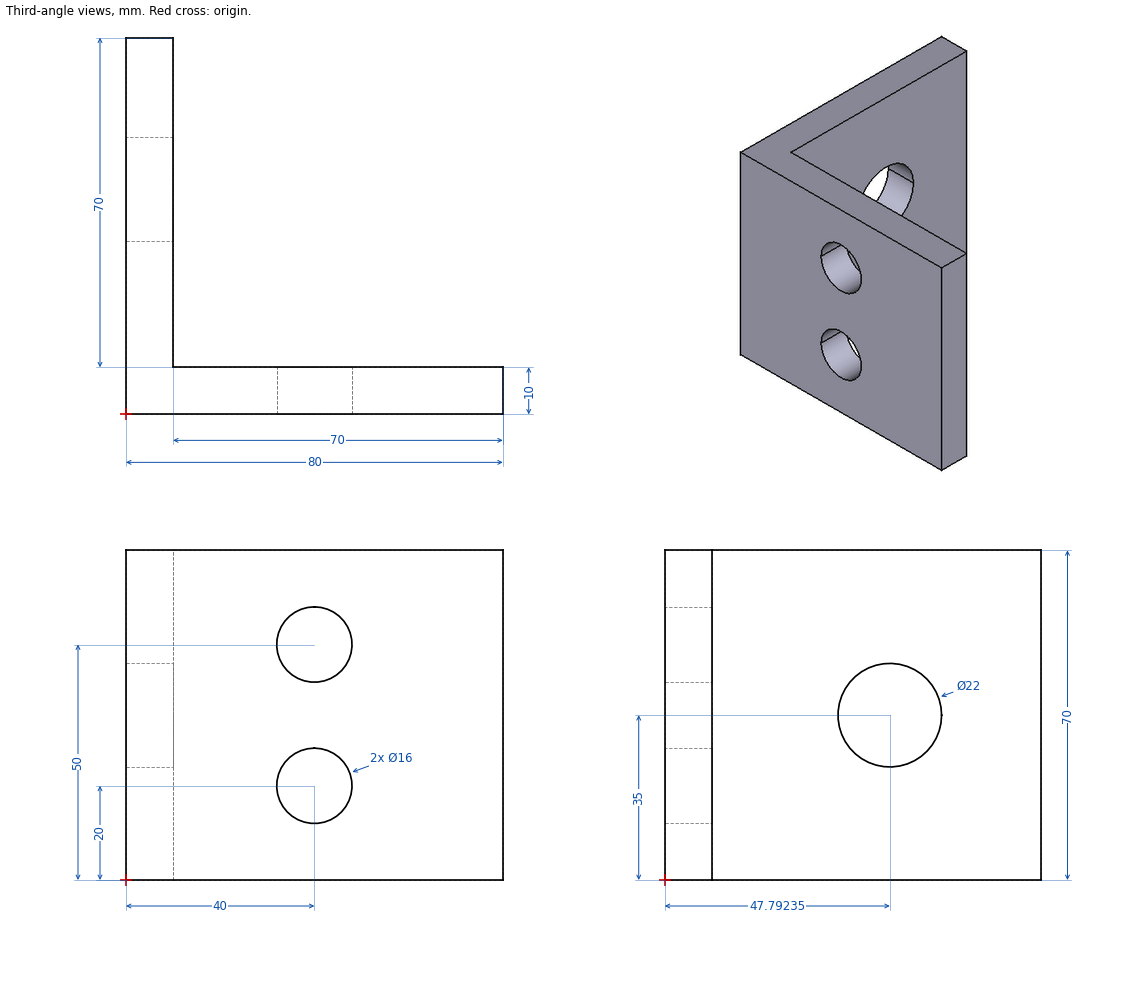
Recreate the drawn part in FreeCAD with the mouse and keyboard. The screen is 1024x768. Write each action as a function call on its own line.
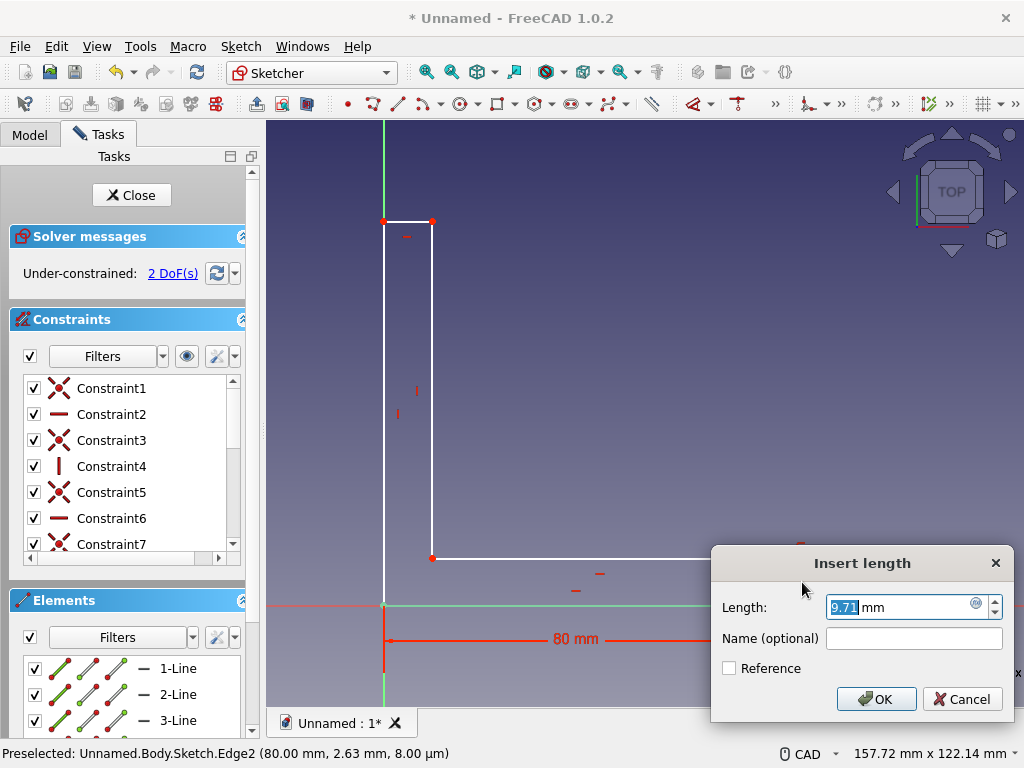
text(10)
key(Return)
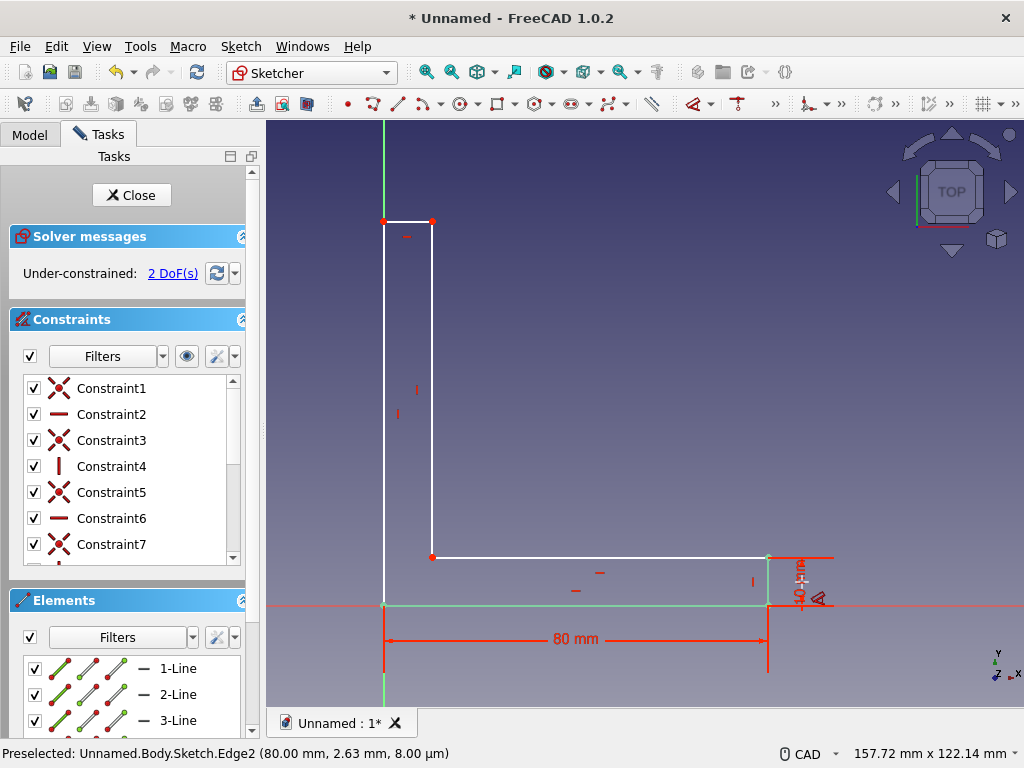
click(667, 558)
click(600, 592)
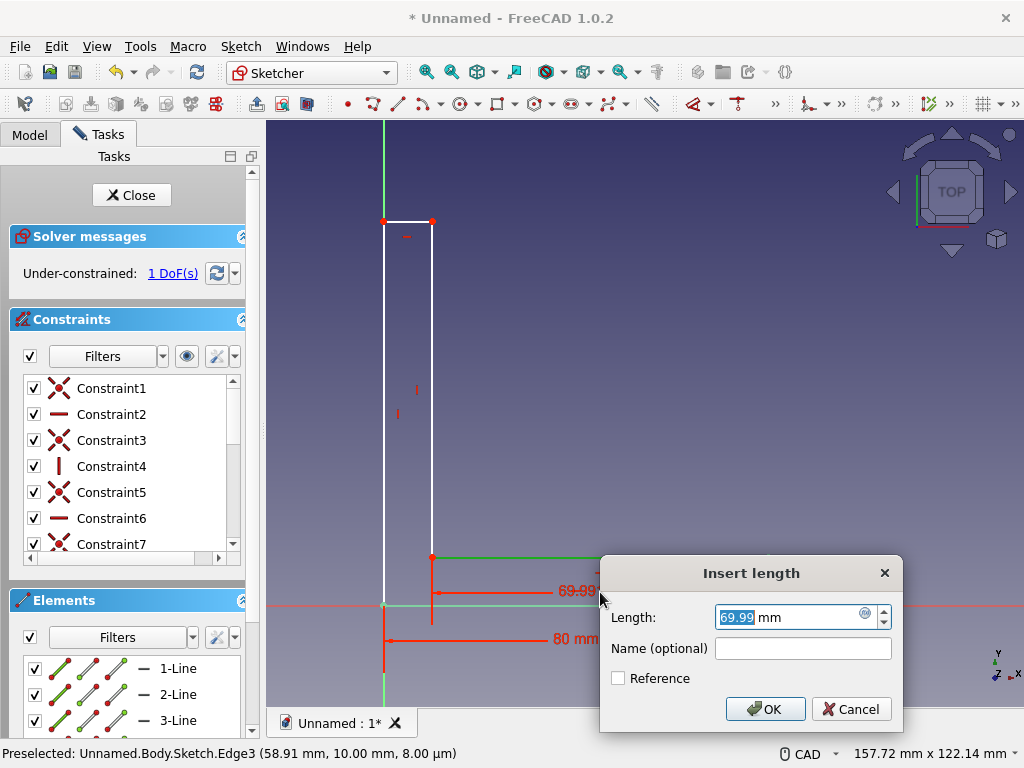
text(70)
key(Return)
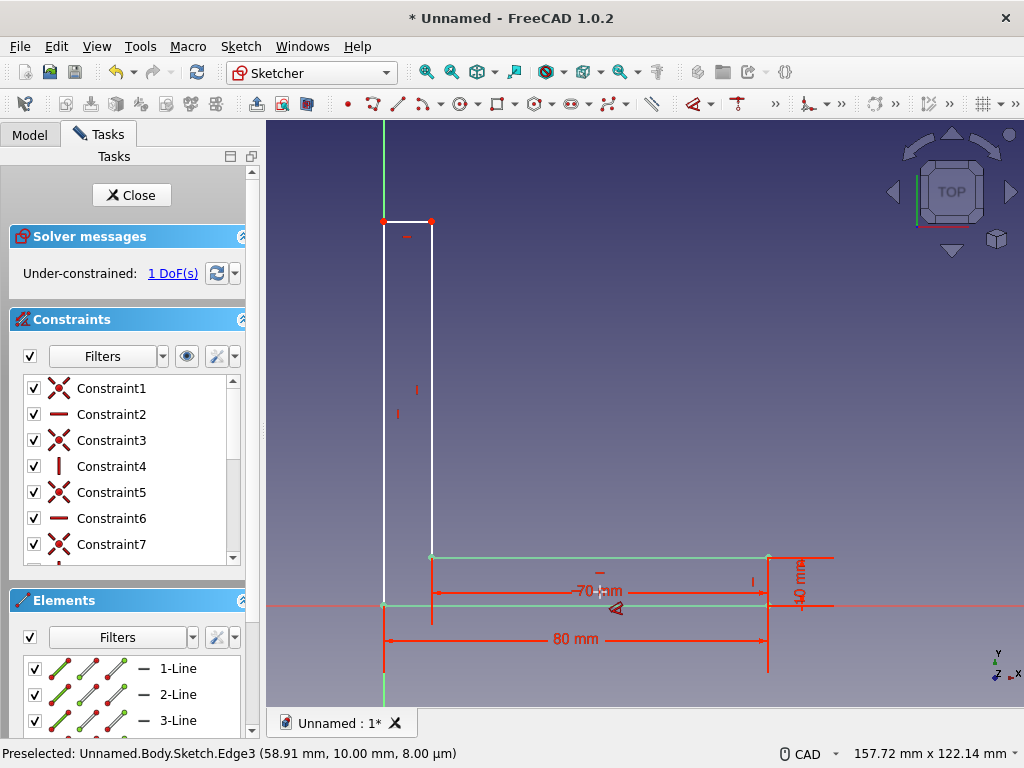
click(432, 457)
click(398, 390)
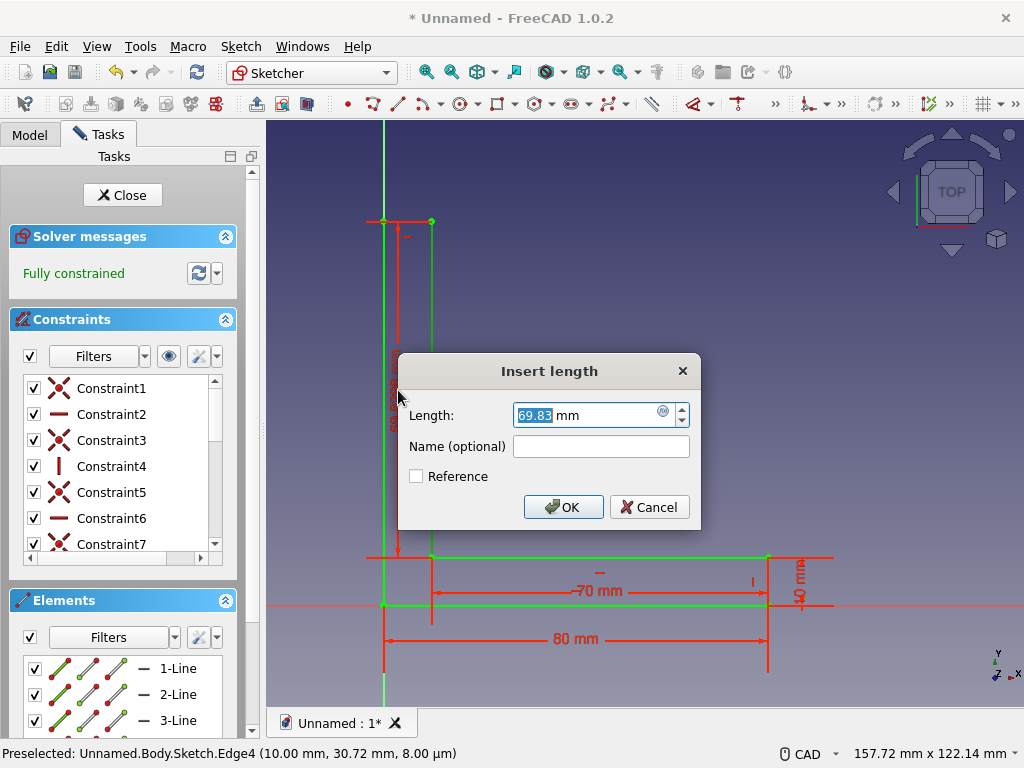
text(70)
key(Return)
key(Escape)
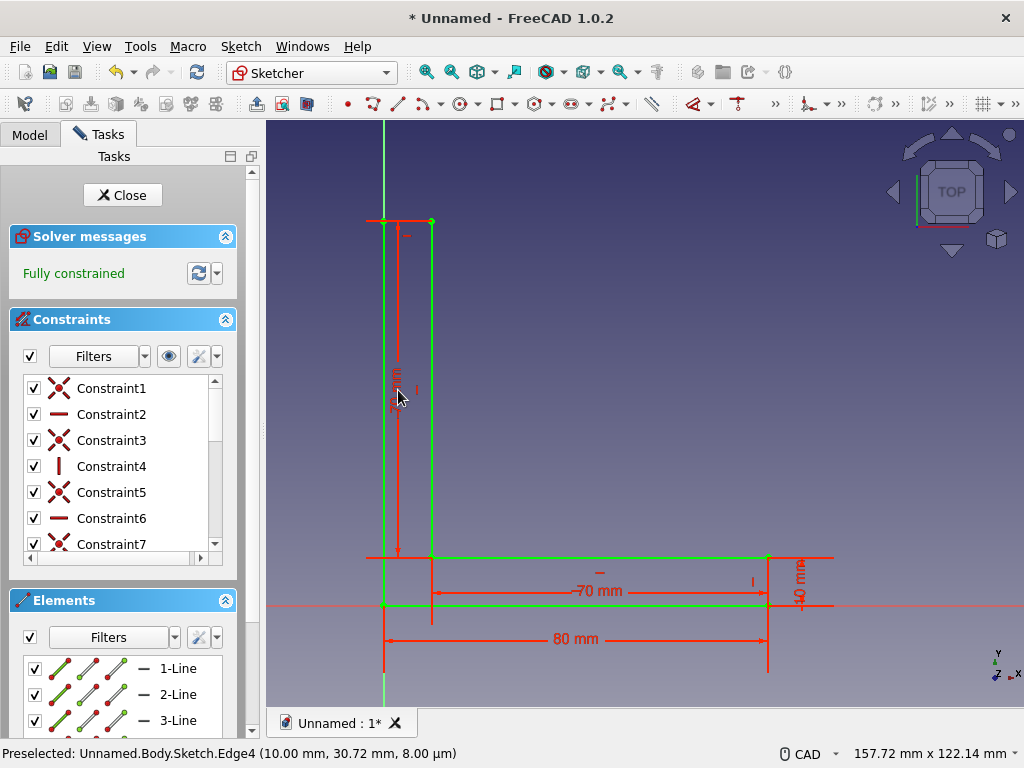
click(123, 195)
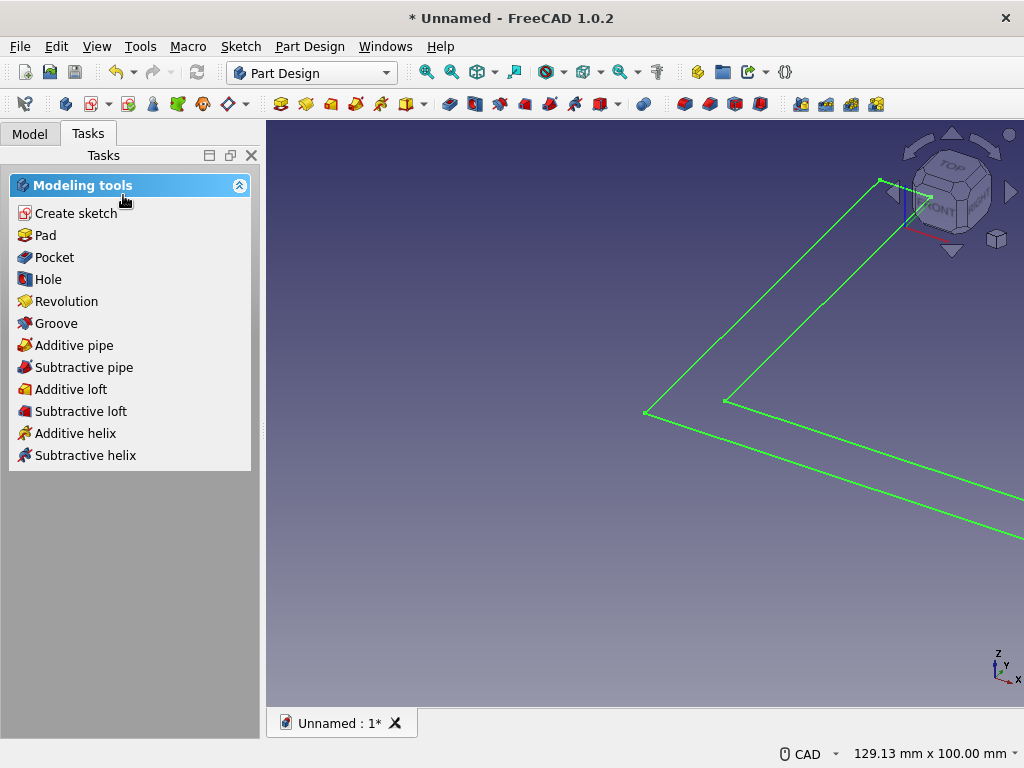
click(281, 104)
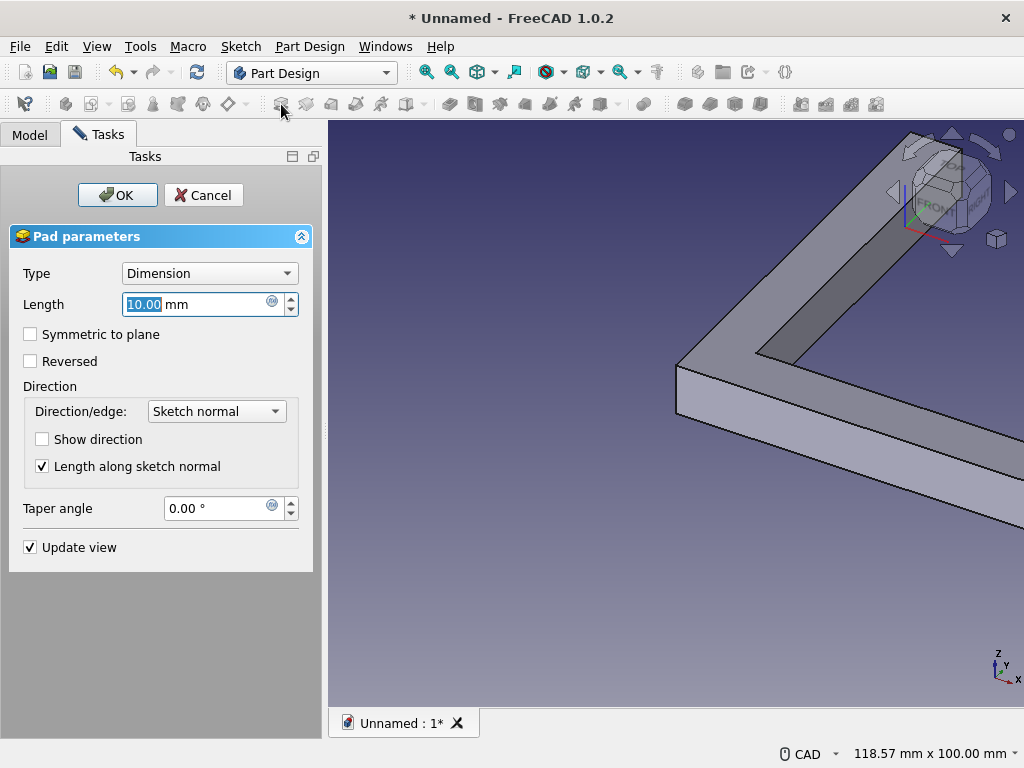
text(70)
key(Tab)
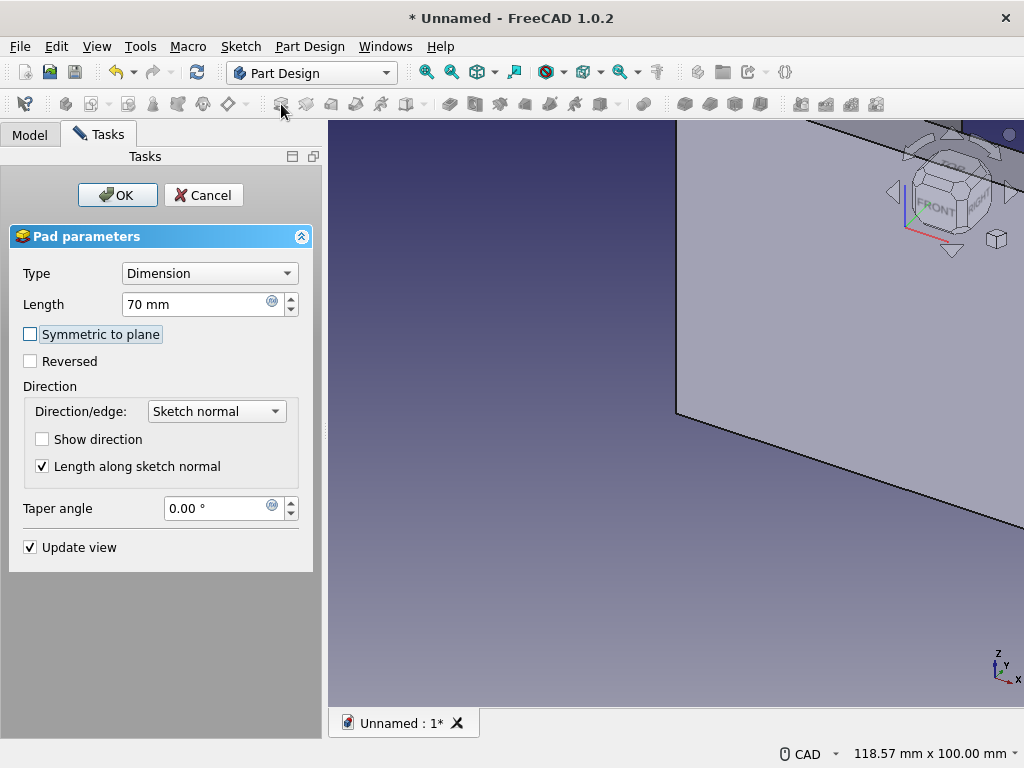
click(118, 195)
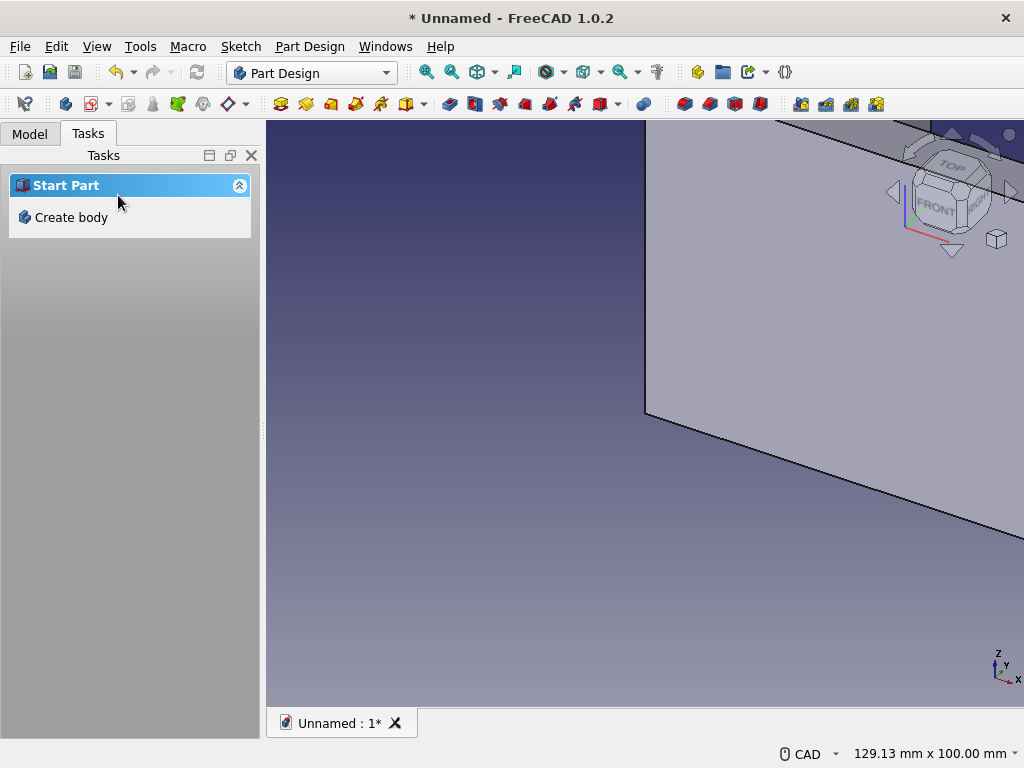
click(427, 72)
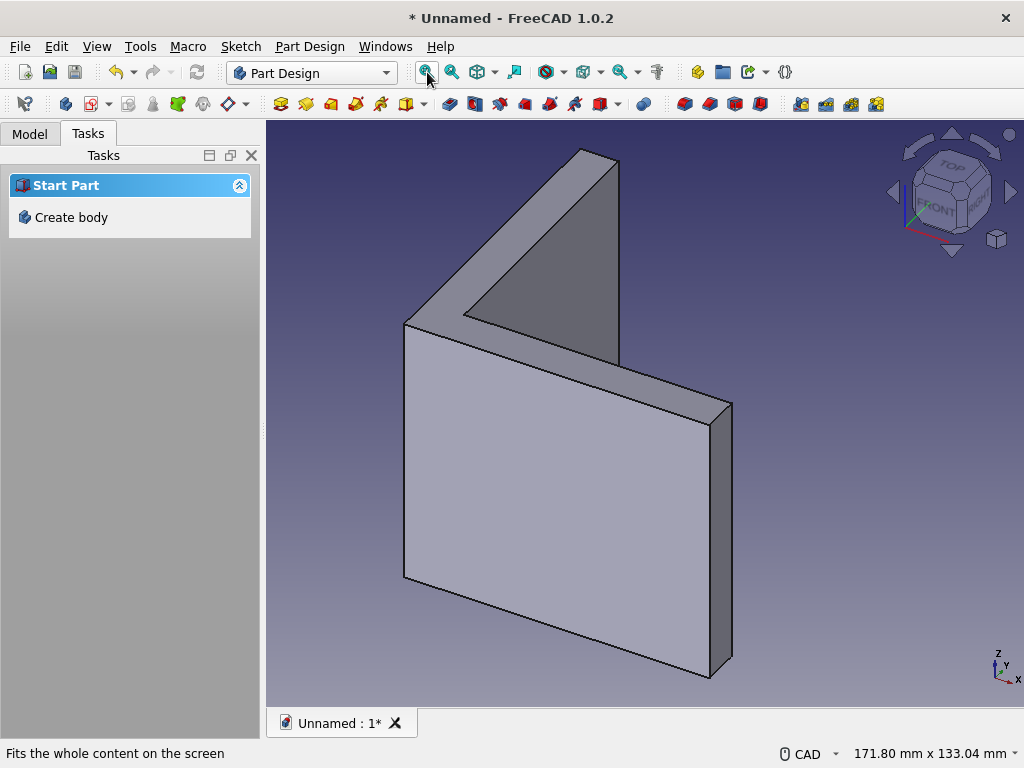
key(4)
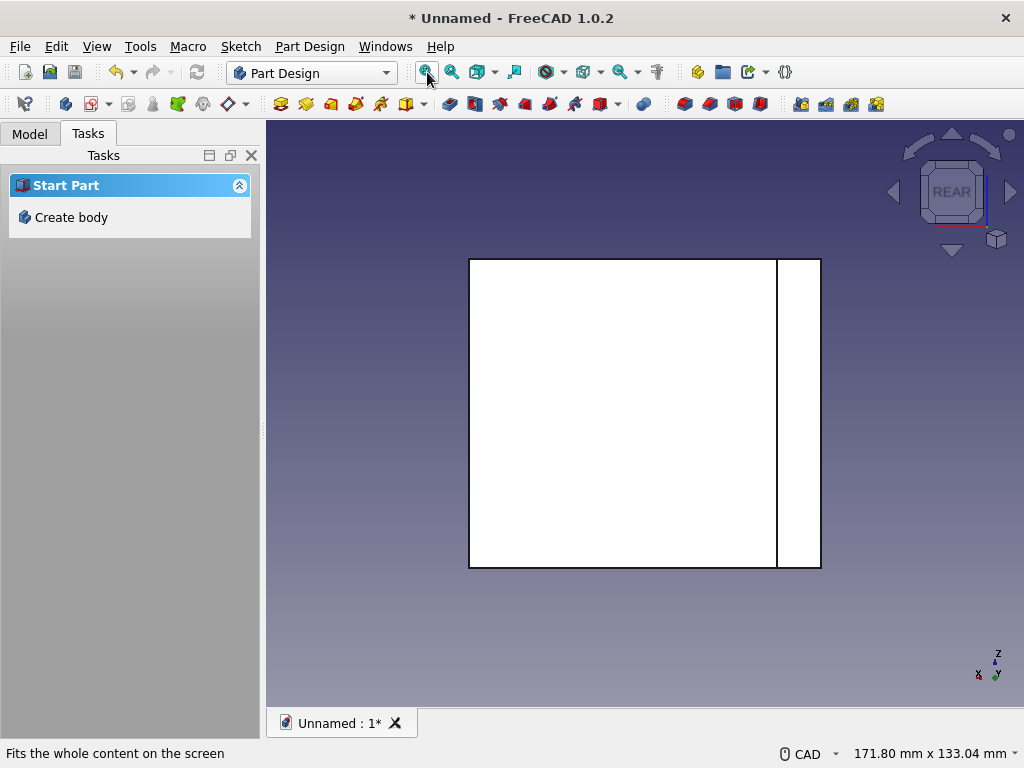
click(623, 412)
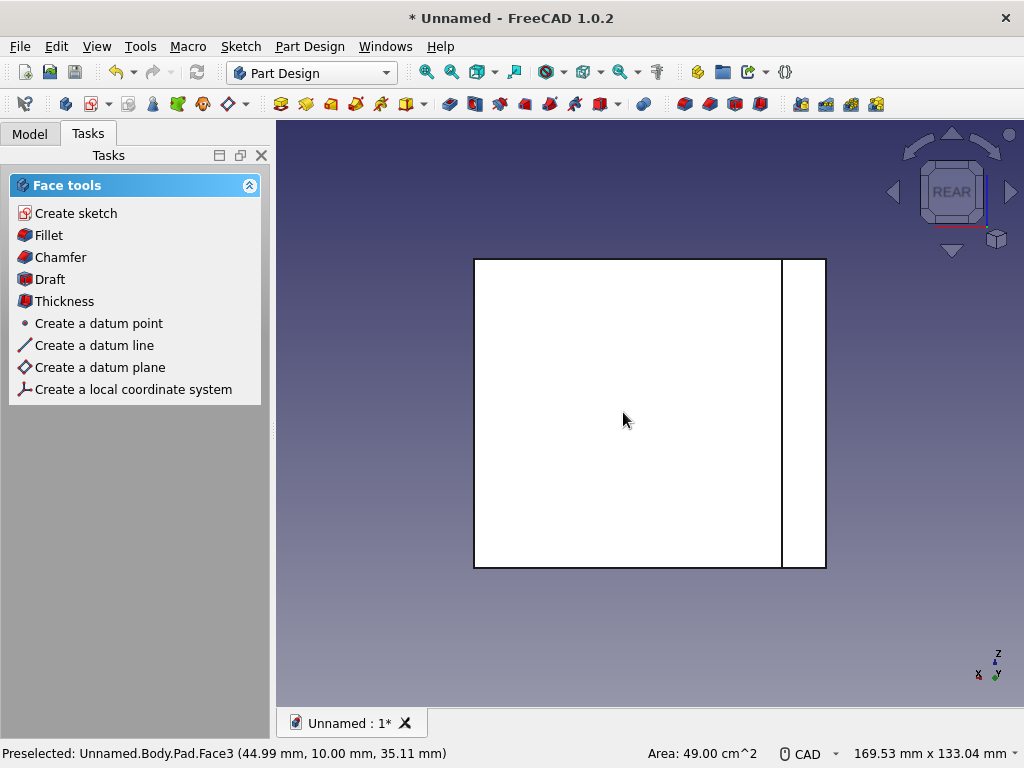
click(90, 104)